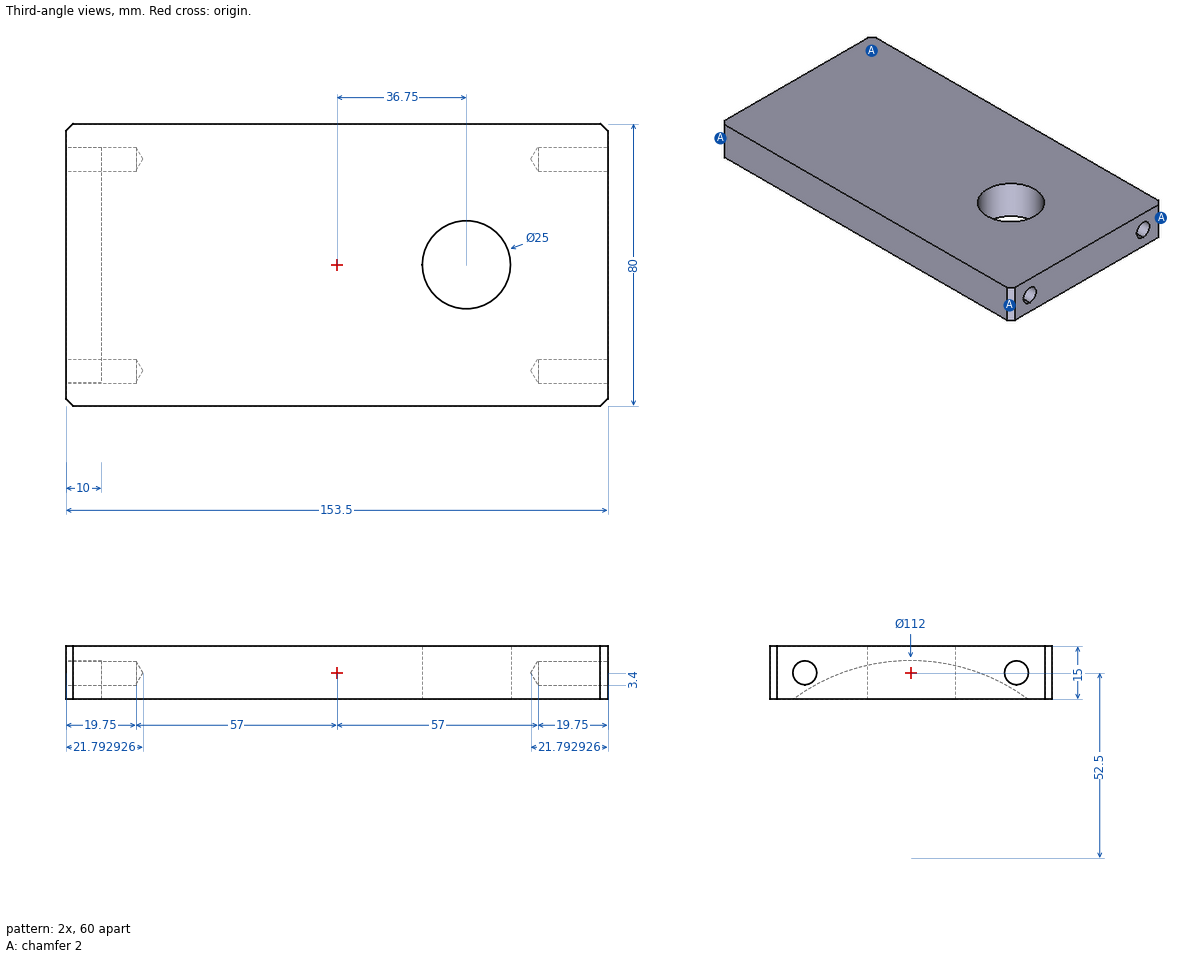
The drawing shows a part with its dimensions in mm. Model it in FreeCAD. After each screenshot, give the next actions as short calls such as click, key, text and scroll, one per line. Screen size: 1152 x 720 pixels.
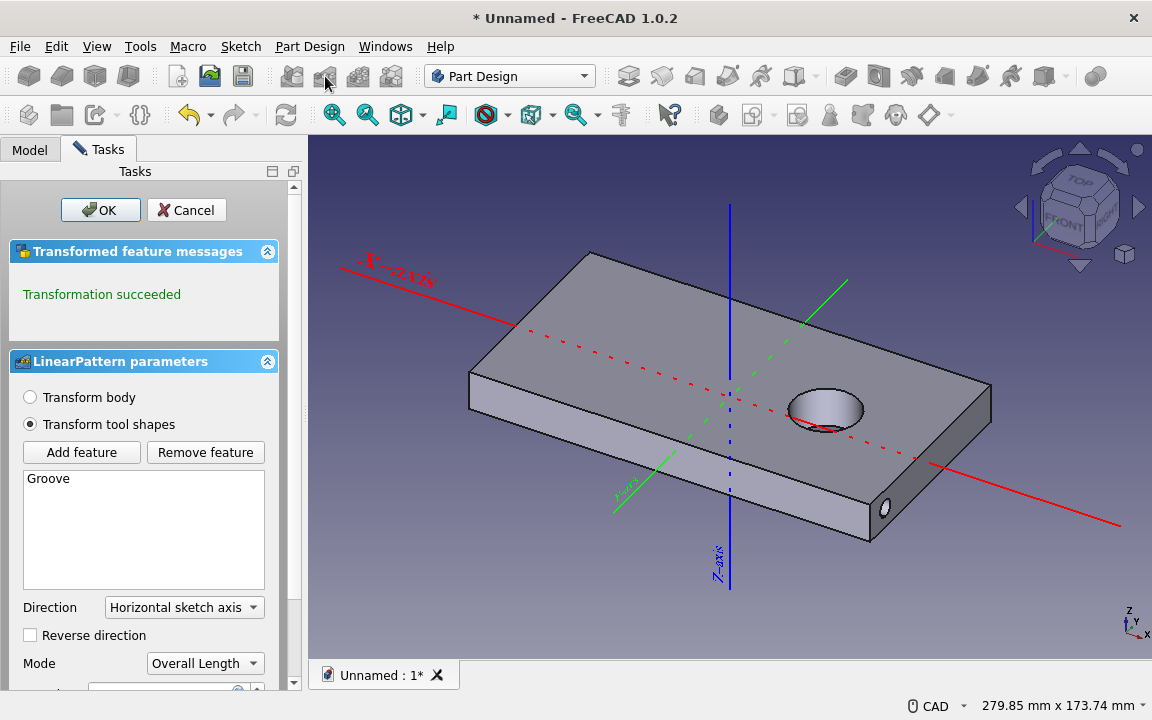
click(185, 608)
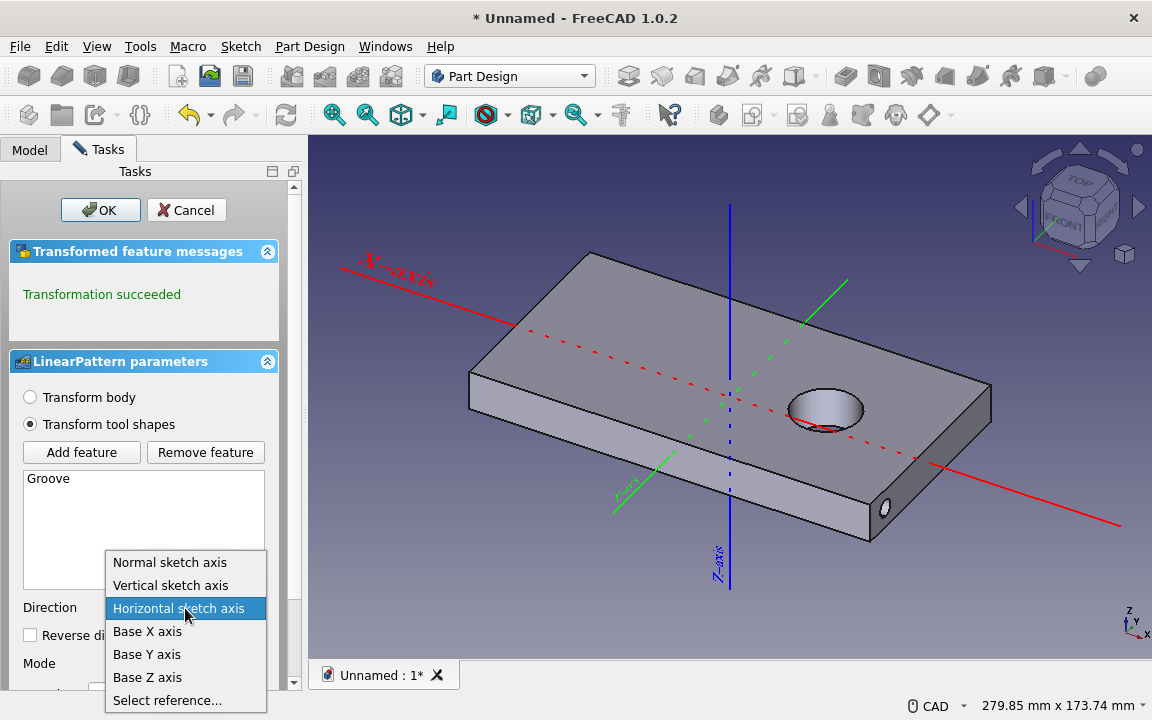
click(184, 654)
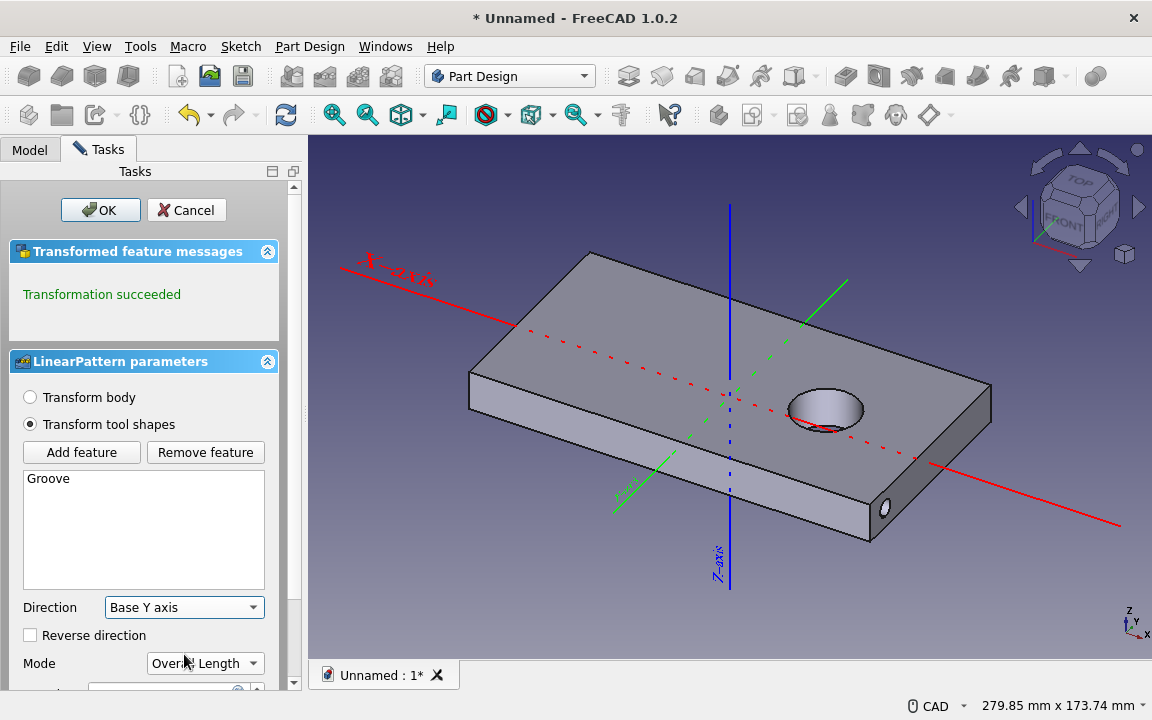
click(206, 664)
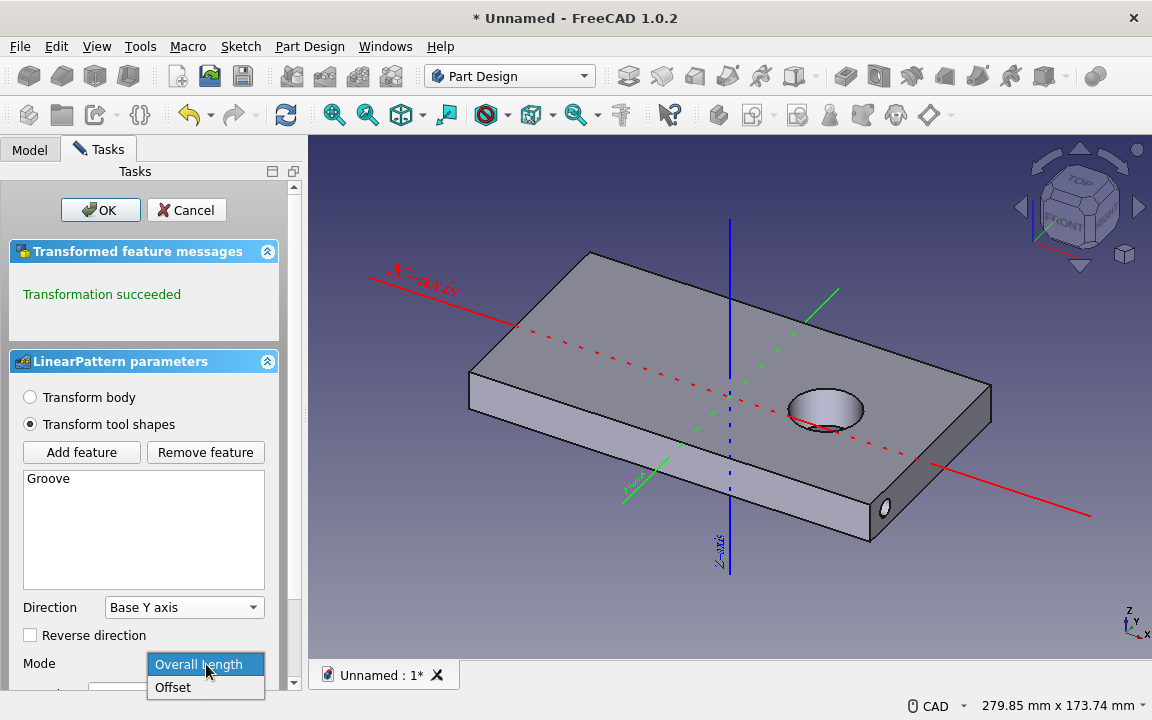
click(204, 688)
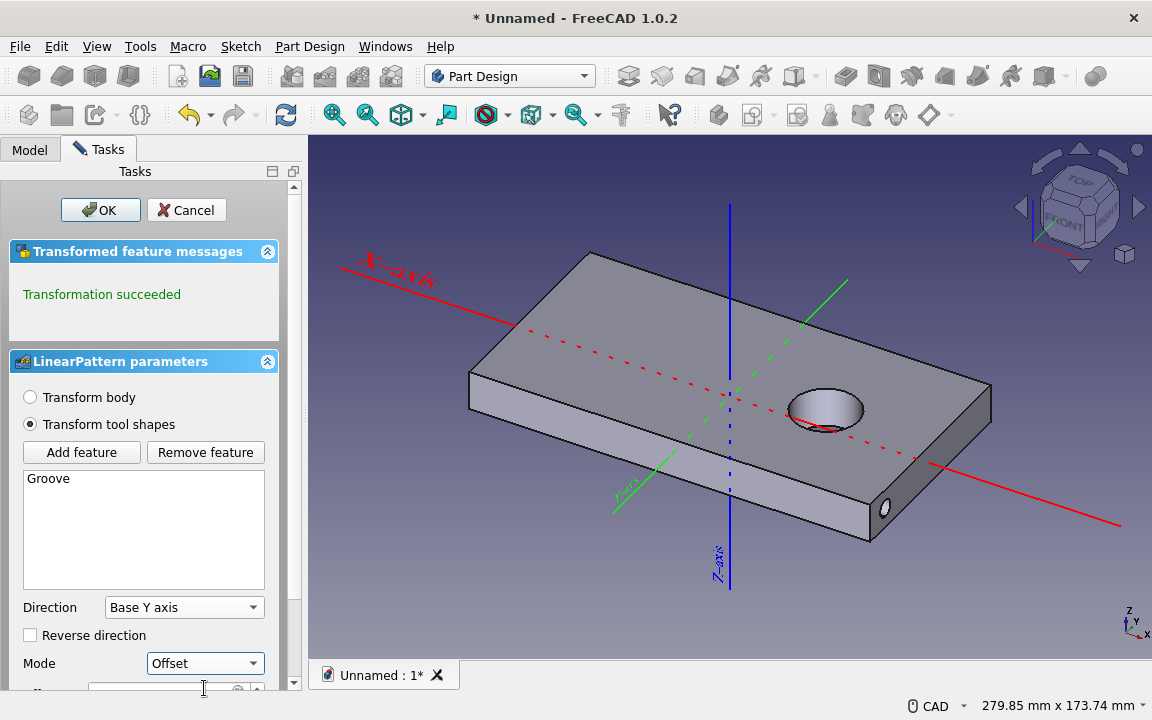
scroll(294, 436, down, 2)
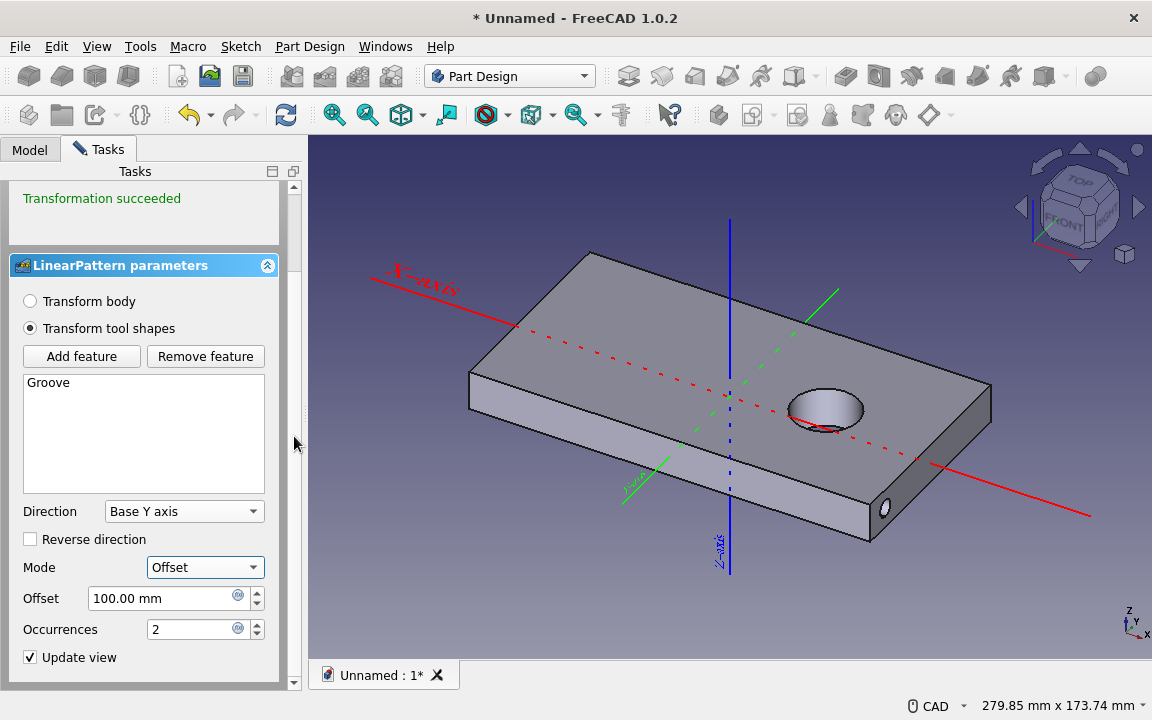
triple_click(170, 598)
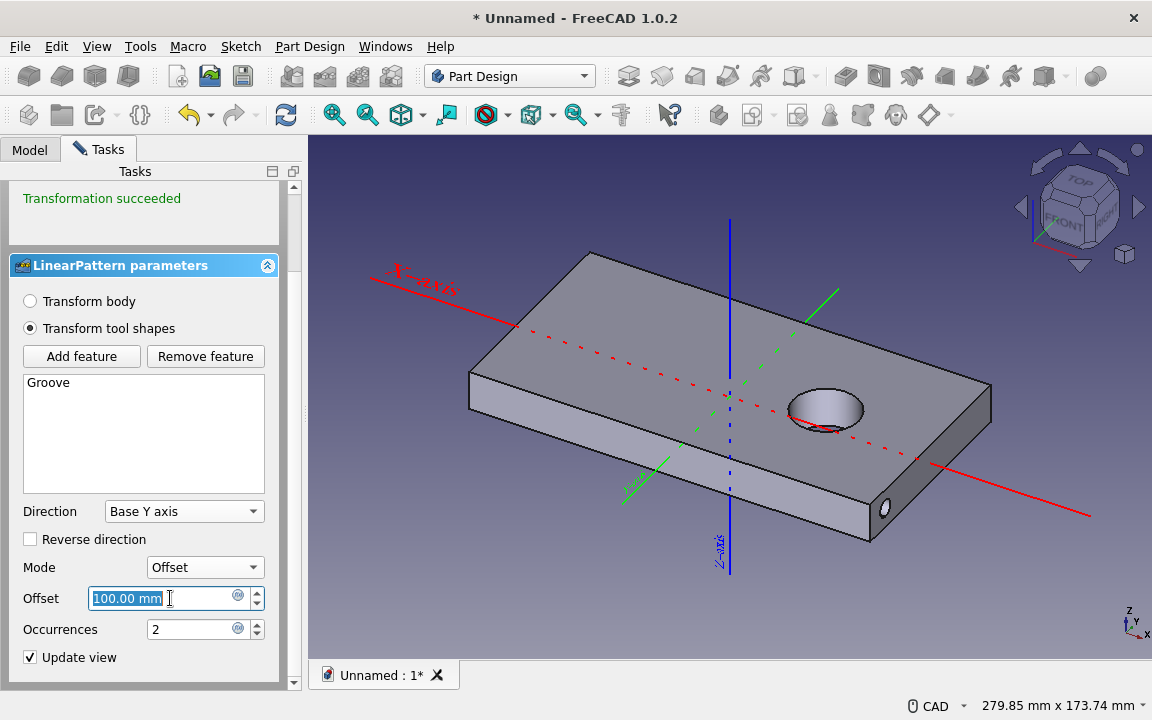
text(60)
key(Tab)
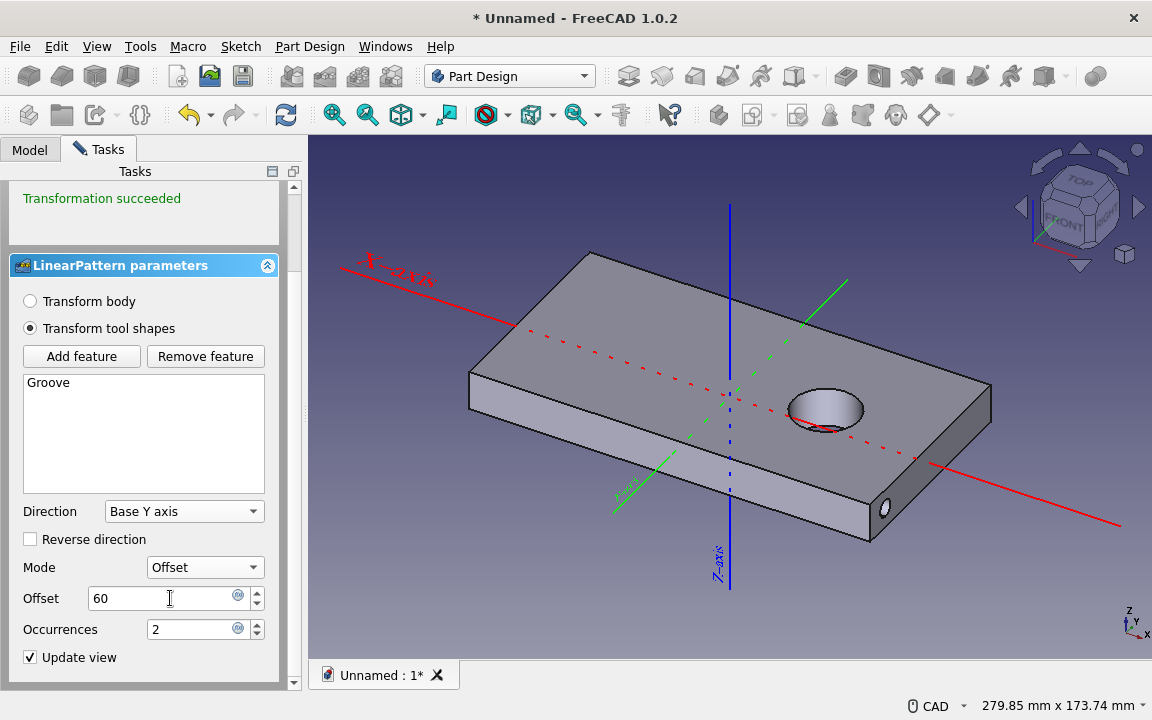
triple_click(199, 630)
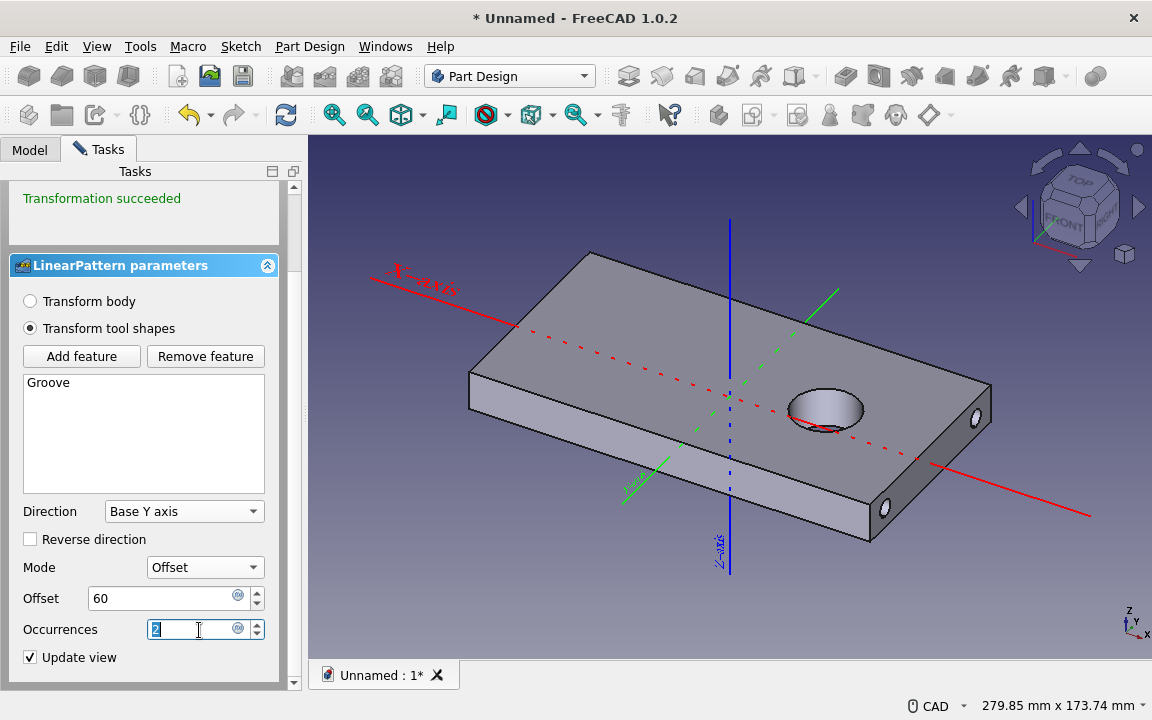
text(2)
key(Tab)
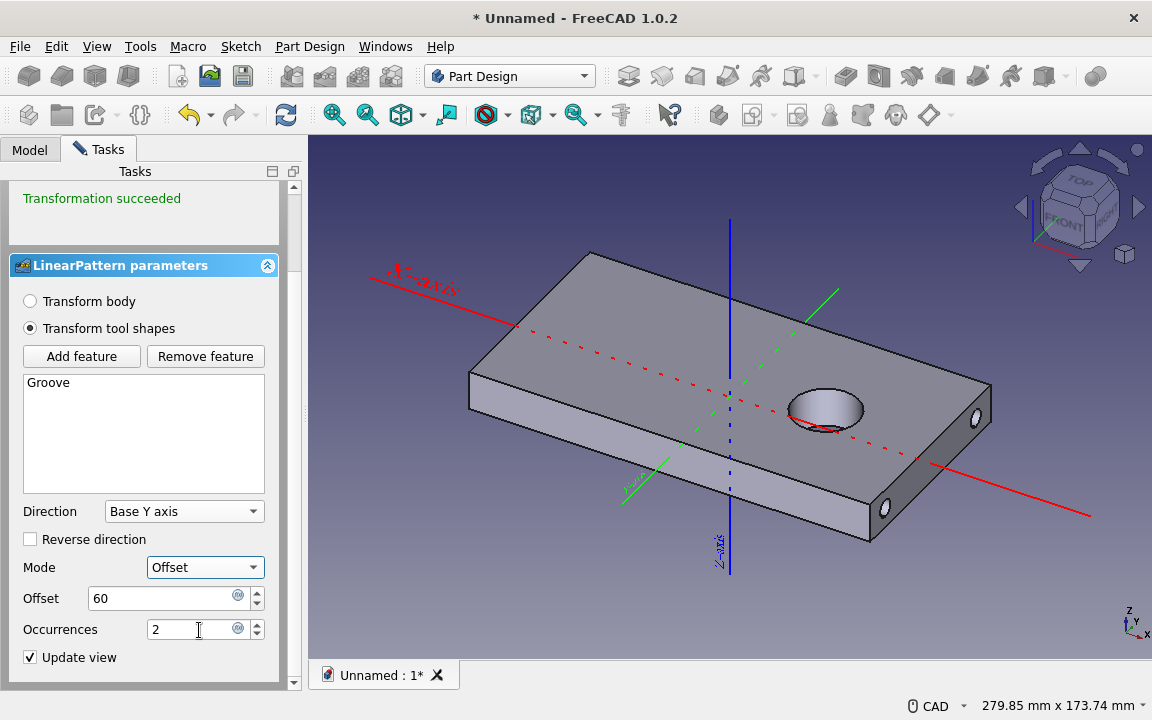
scroll(294, 436, up, 3)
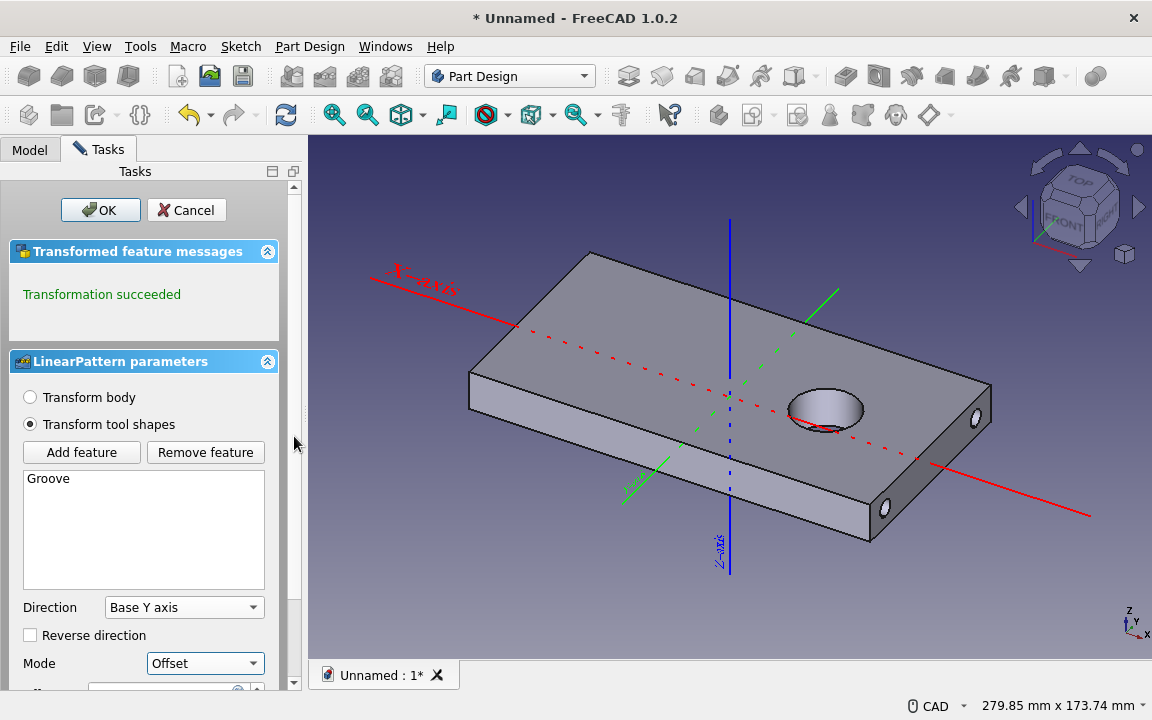
click(101, 210)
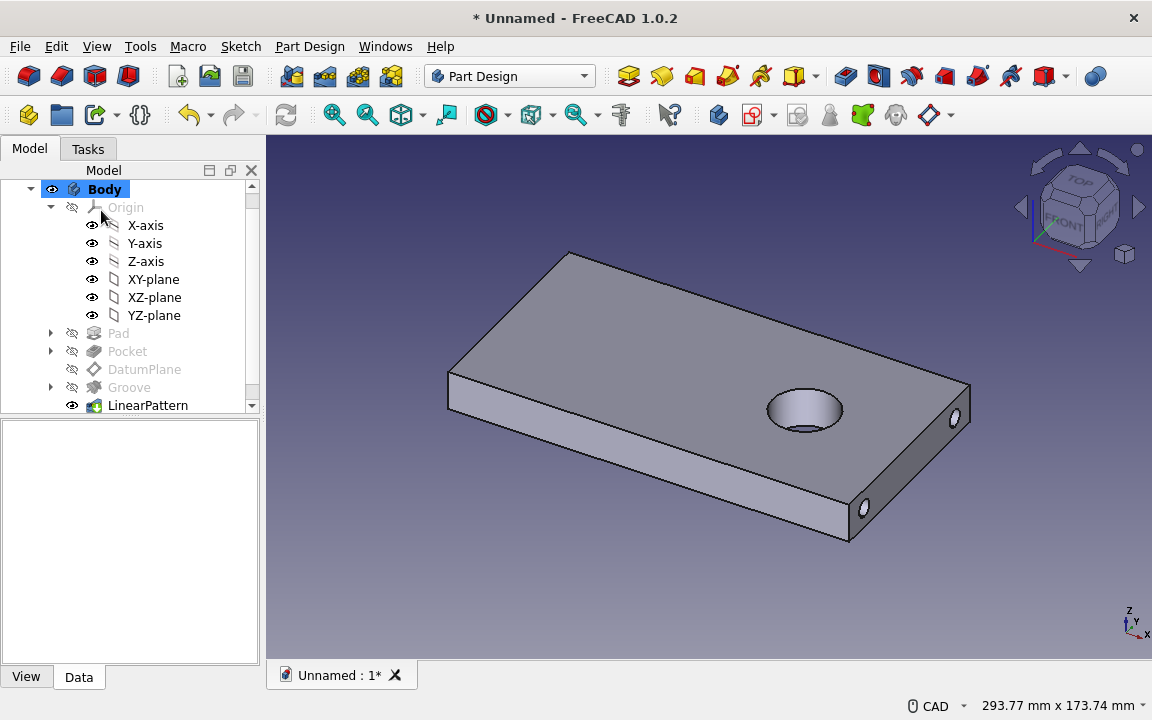
click(117, 387)